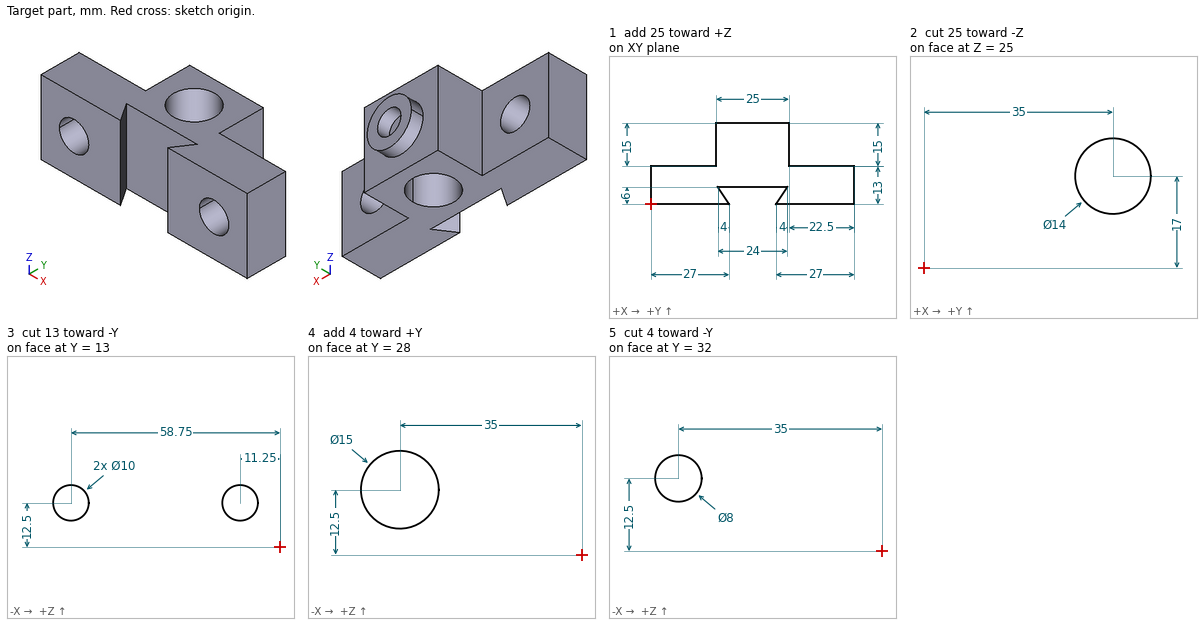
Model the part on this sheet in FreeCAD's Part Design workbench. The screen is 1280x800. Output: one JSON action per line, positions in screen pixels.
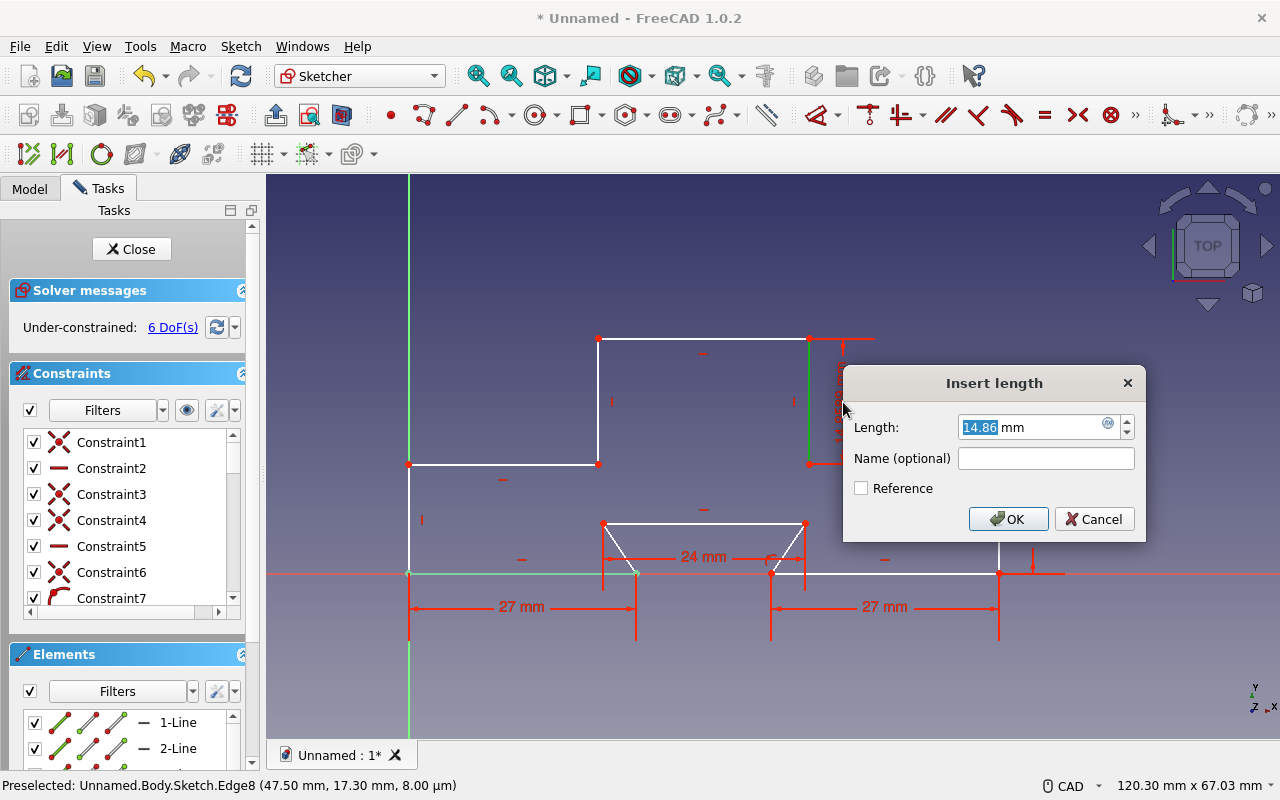
{"action": "type", "text": "15"}
{"action": "key", "text": "Return"}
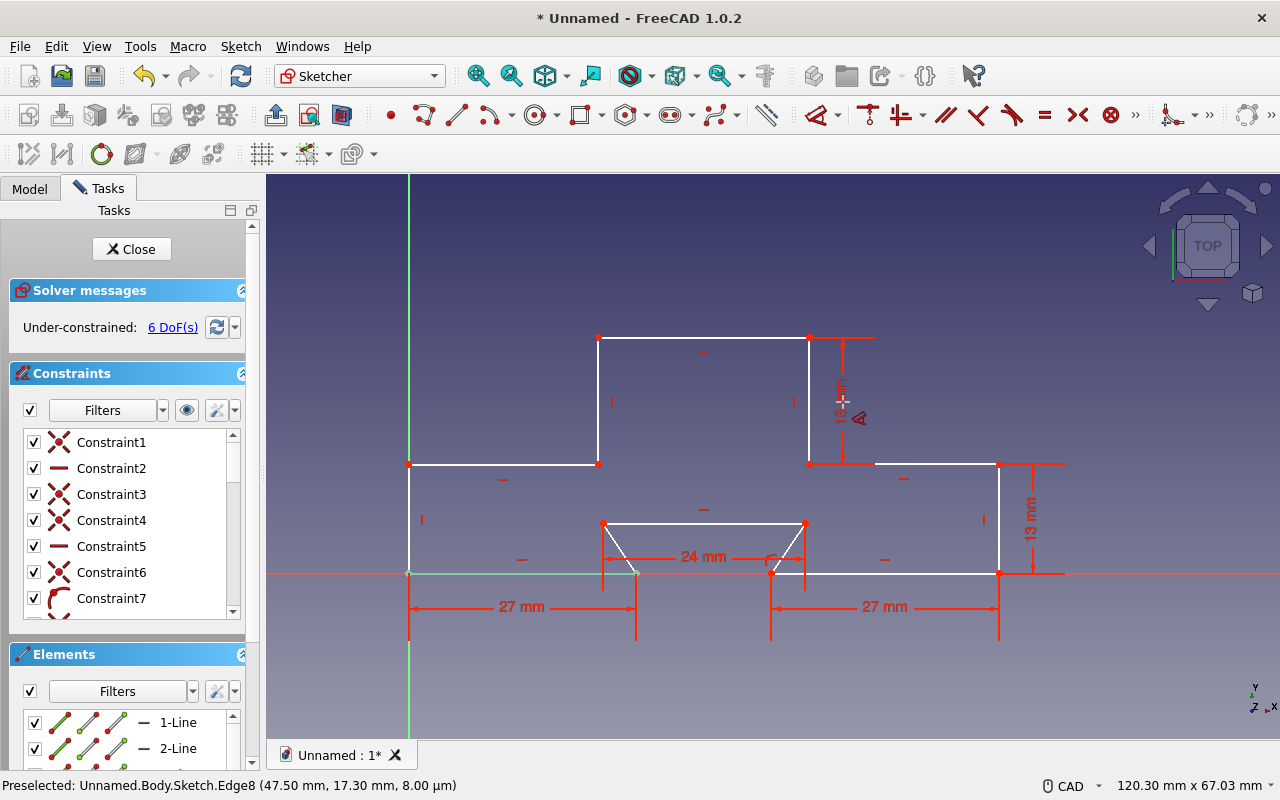
{"action": "left_click", "coordinate": [746, 338]}
{"action": "left_click", "coordinate": [704, 304]}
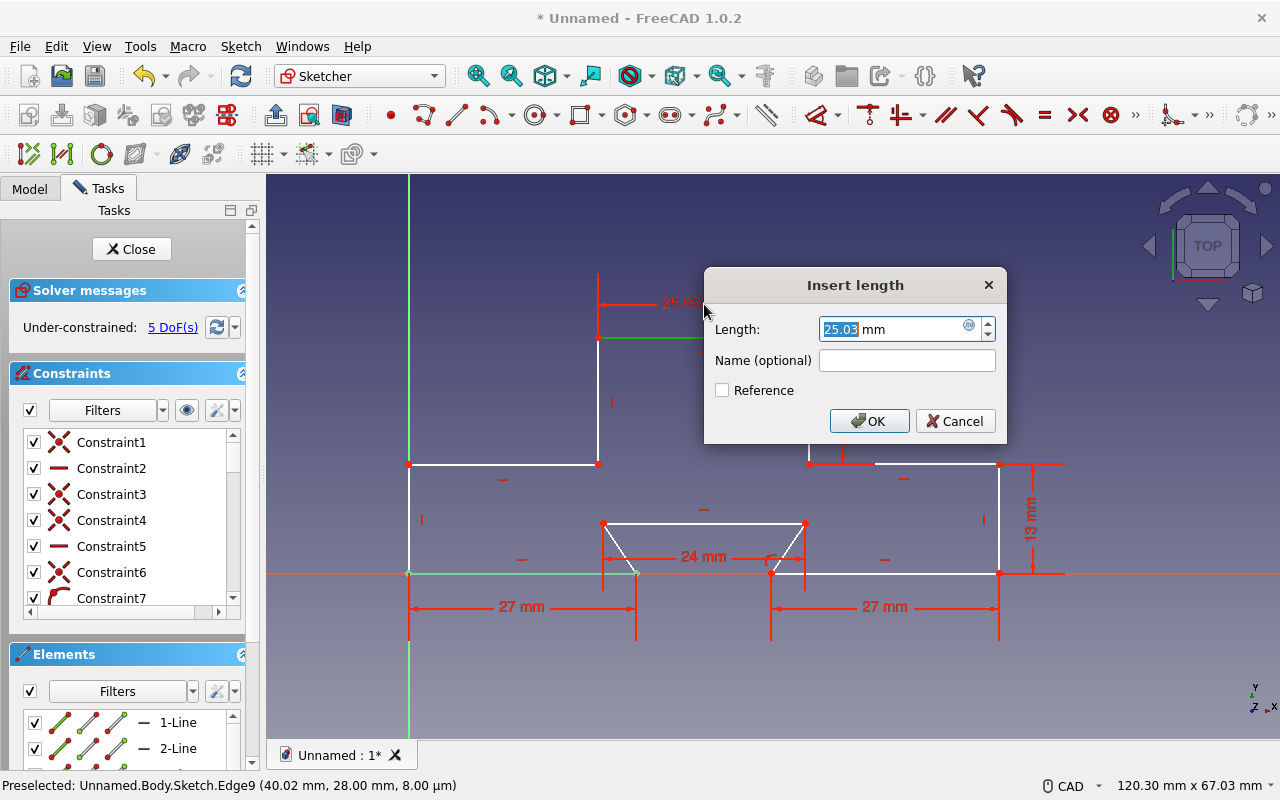
{"action": "type", "text": "25"}
{"action": "key", "text": "Return"}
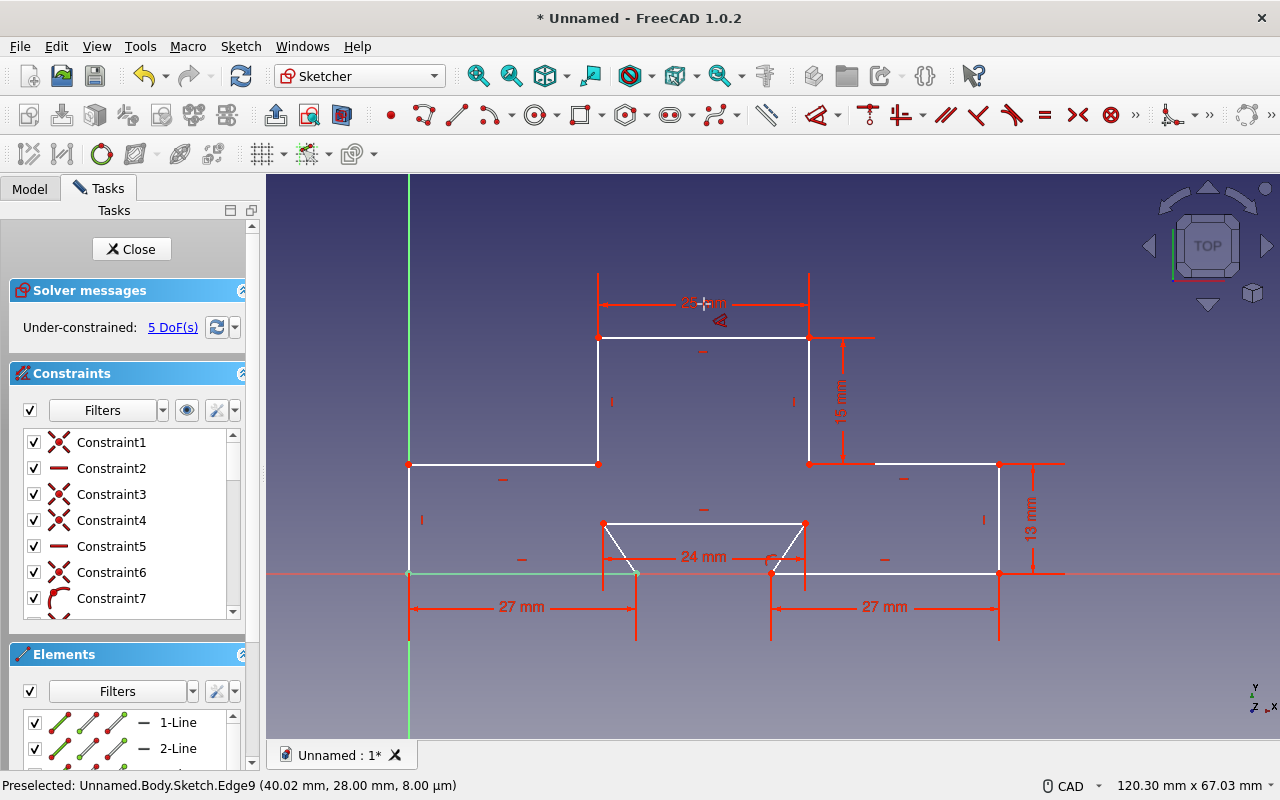
{"action": "left_click", "coordinate": [598, 376]}
{"action": "left_click", "coordinate": [564, 401]}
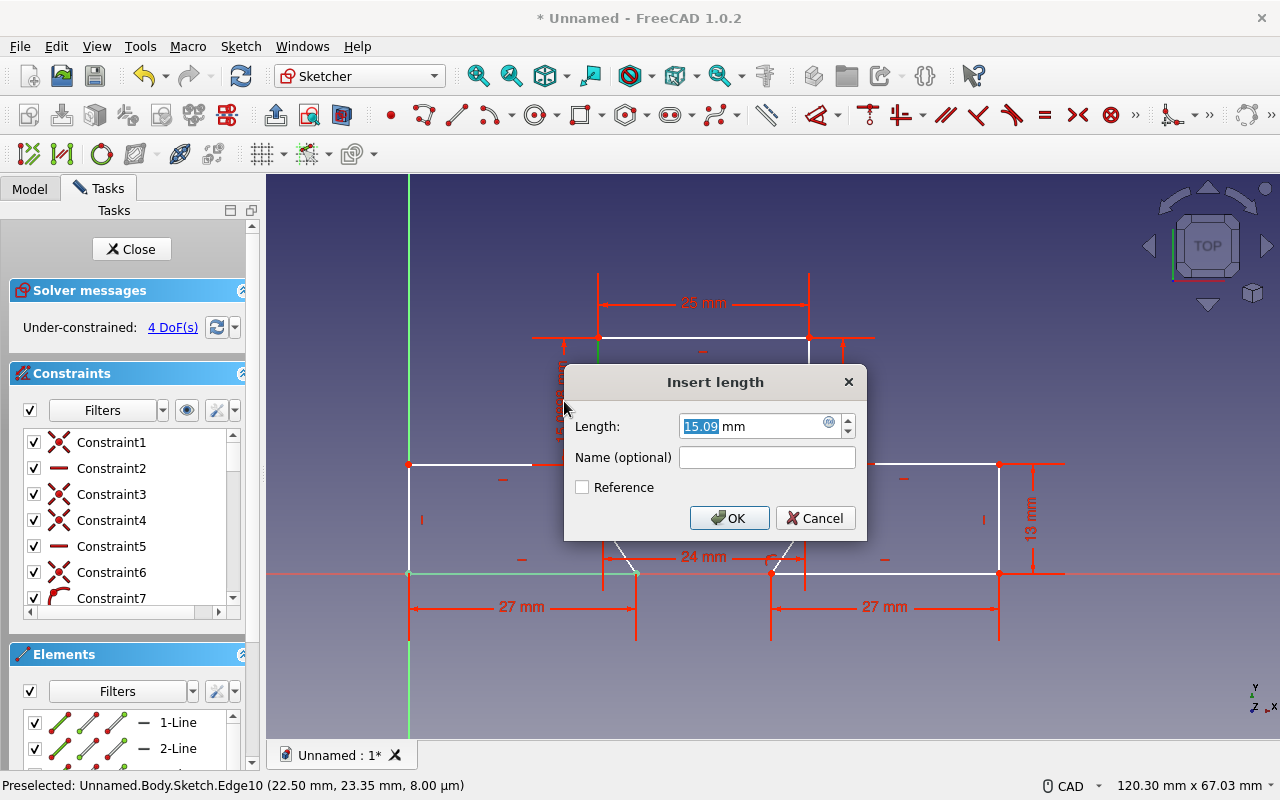
{"action": "type", "text": "15"}
{"action": "key", "text": "Return"}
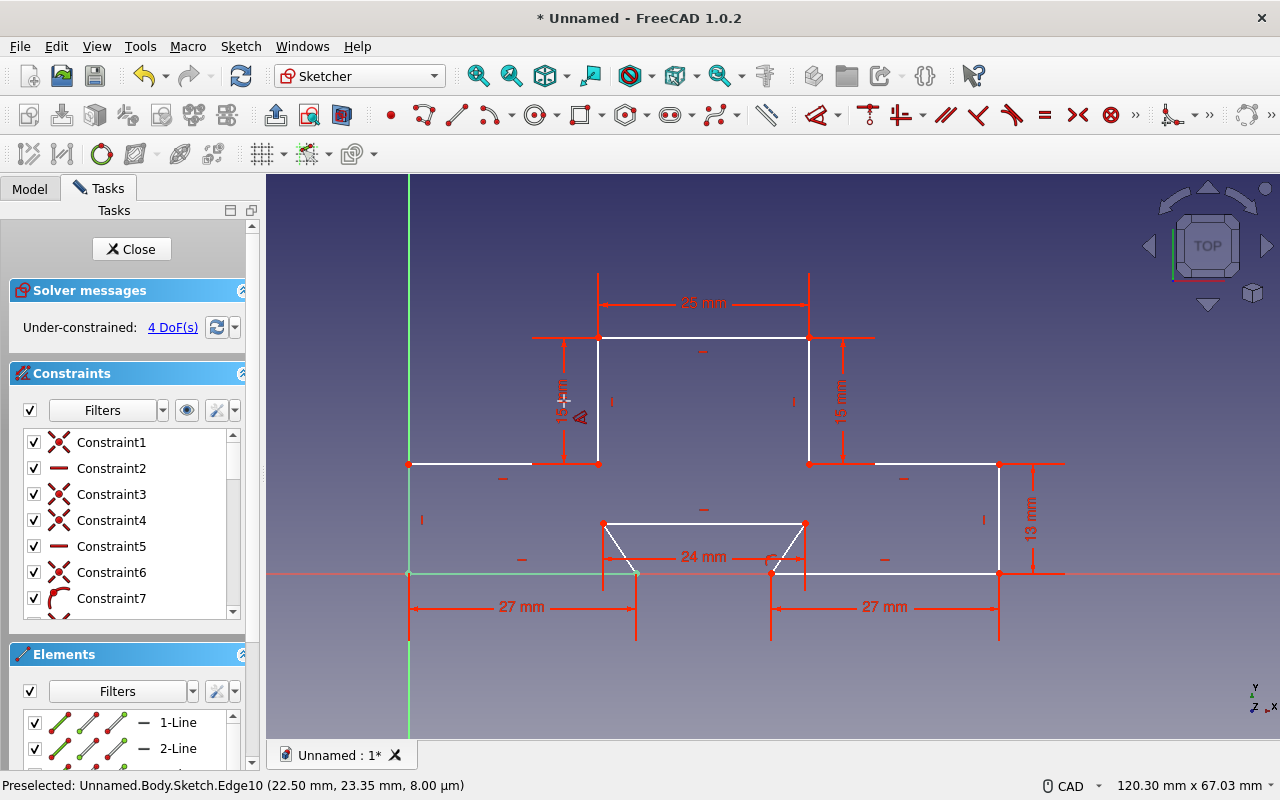
{"action": "left_click", "coordinate": [603, 524]}
{"action": "left_click", "coordinate": [375, 549]}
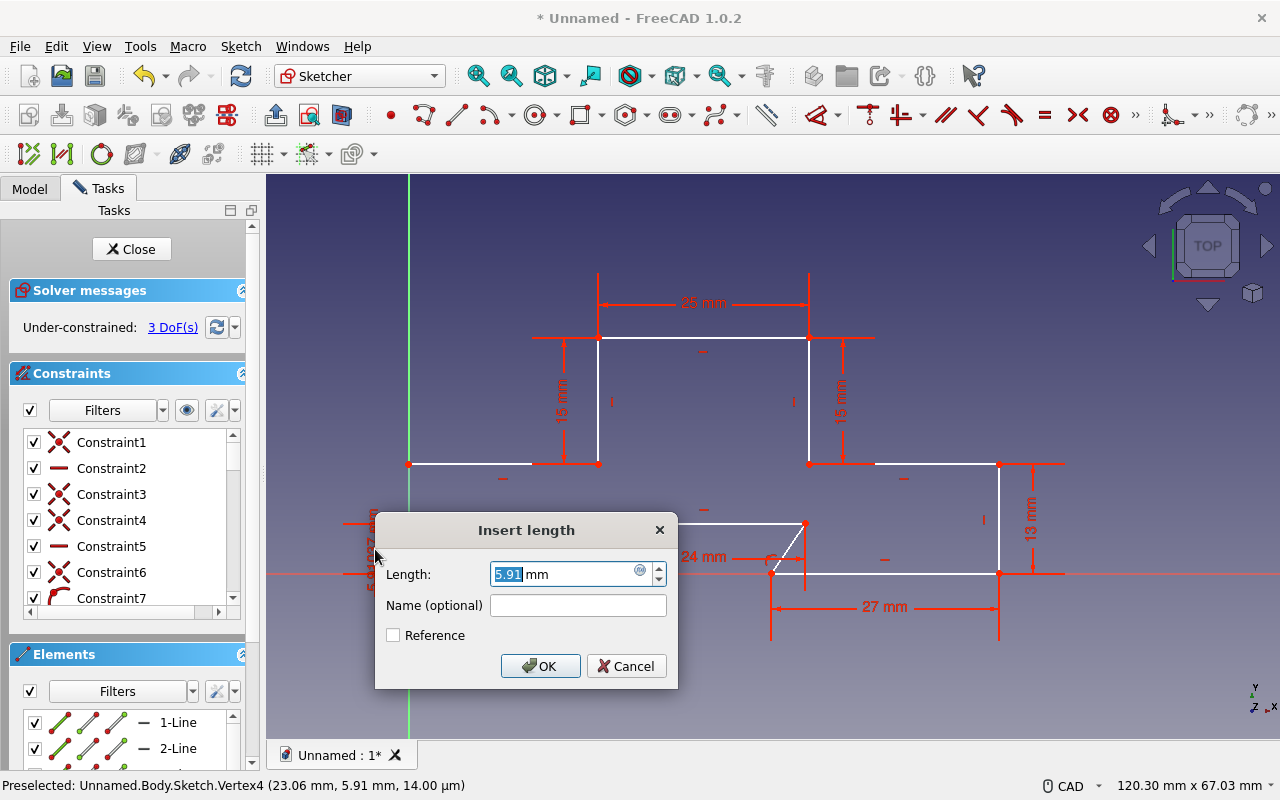
{"action": "type", "text": "6"}
{"action": "key", "text": "Return"}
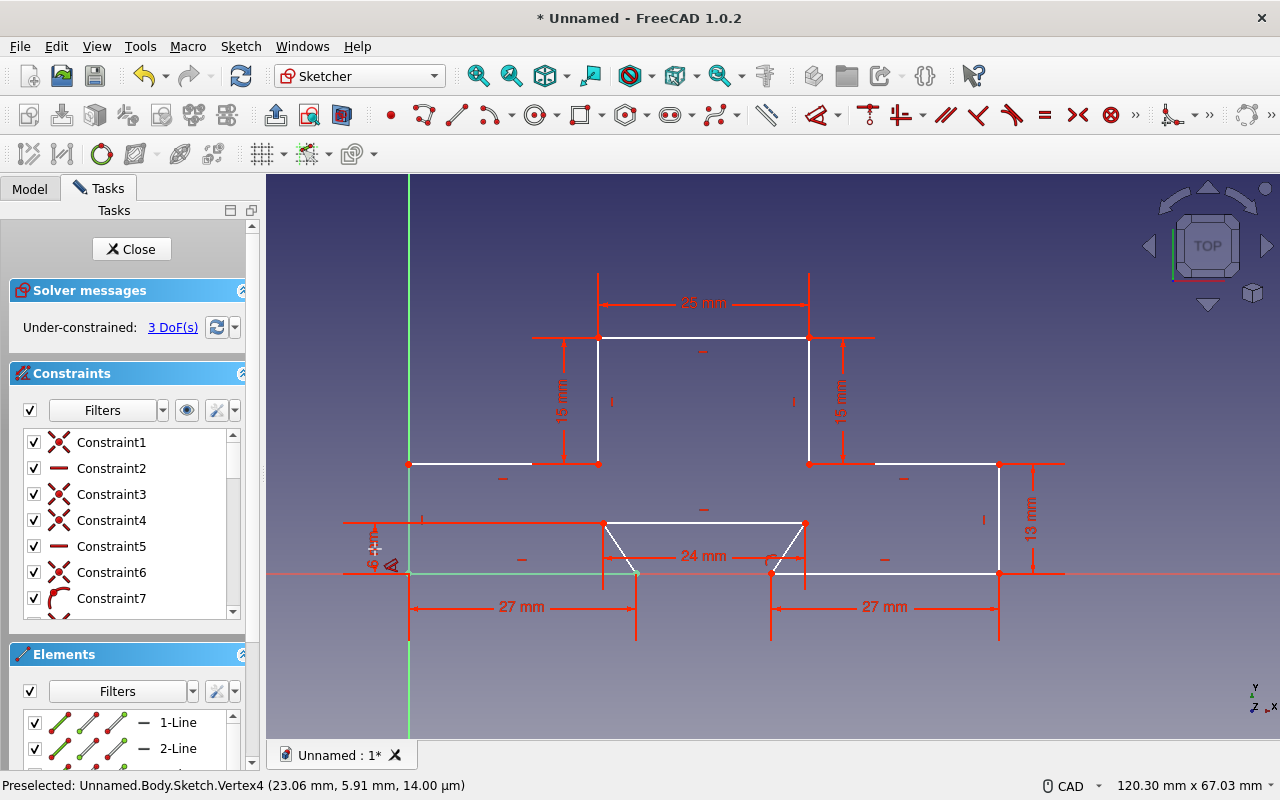
{"action": "left_click", "coordinate": [626, 559]}
{"action": "left_click", "coordinate": [620, 608]}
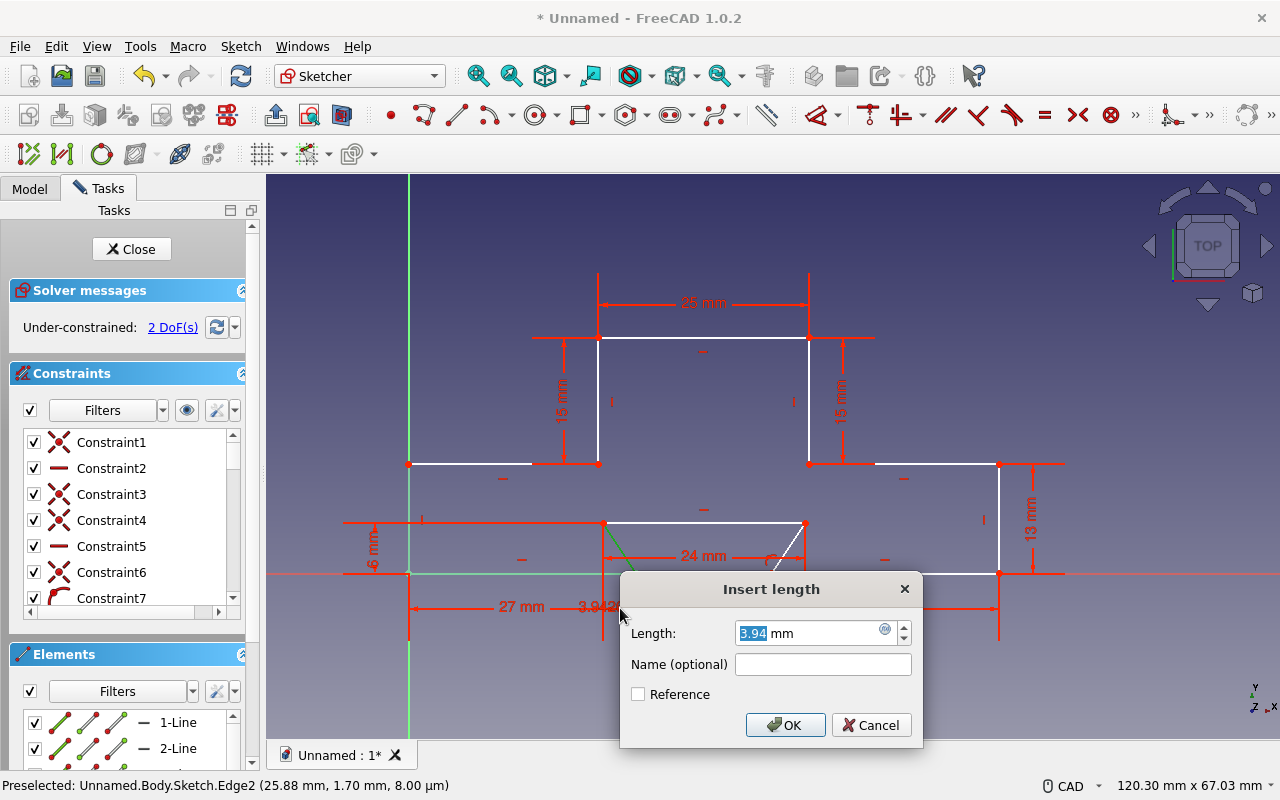
{"action": "type", "text": "4"}
{"action": "key", "text": "Return"}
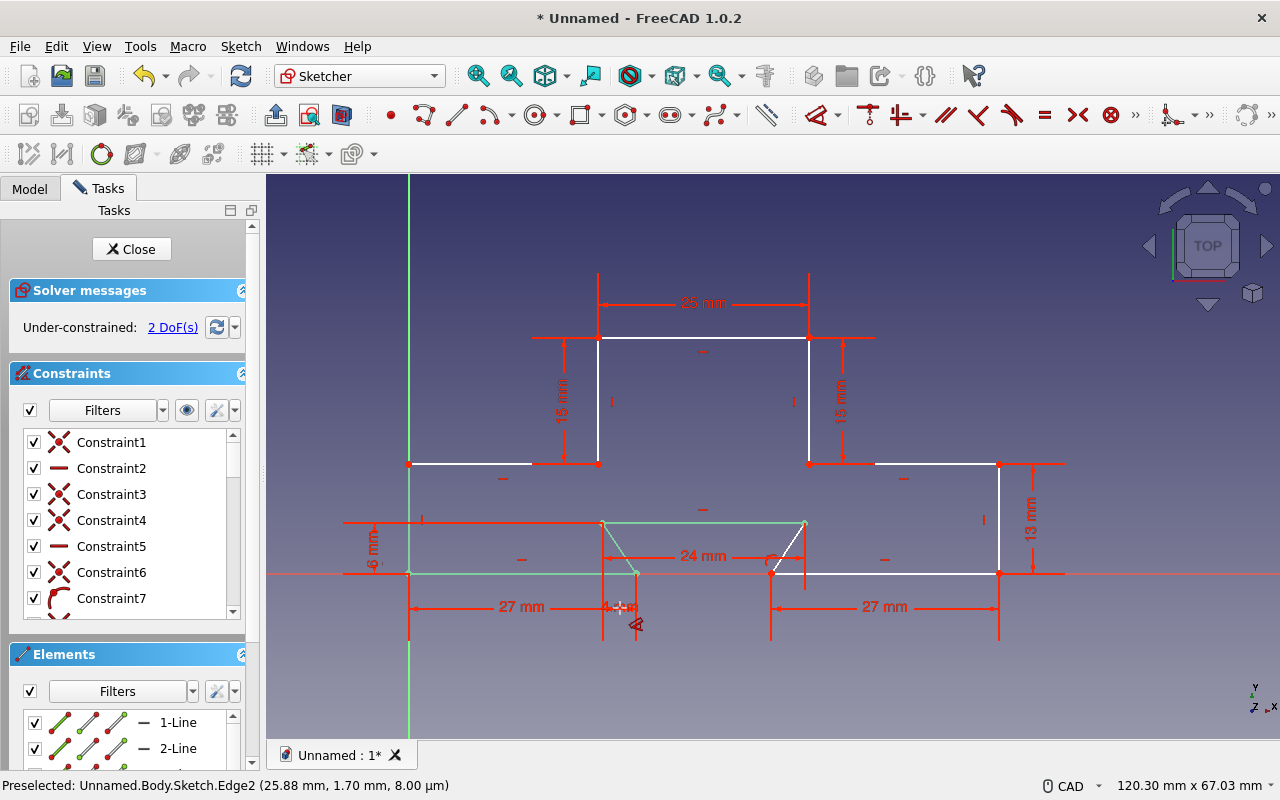
{"action": "left_click", "coordinate": [795, 538]}
{"action": "left_click", "coordinate": [788, 608]}